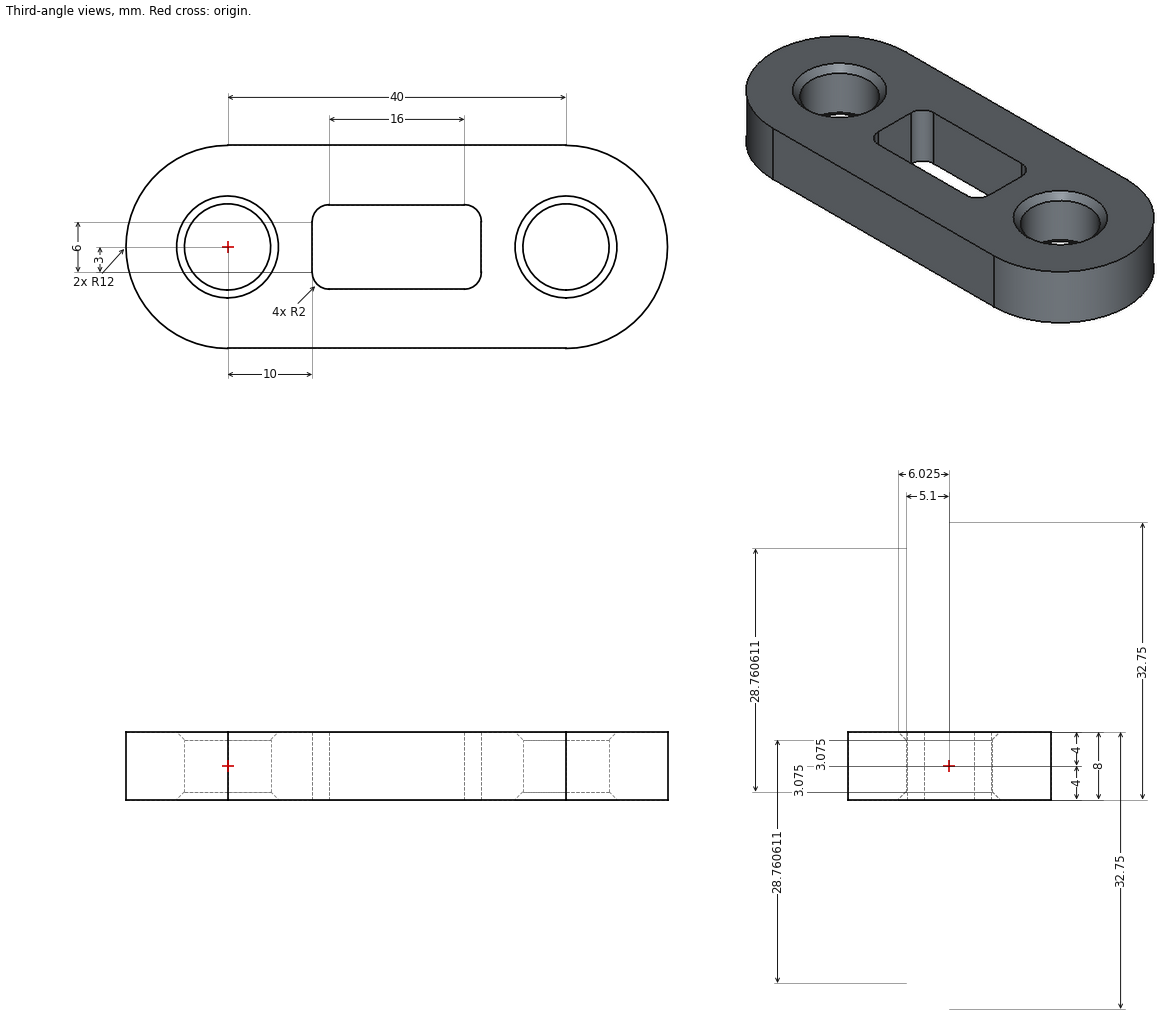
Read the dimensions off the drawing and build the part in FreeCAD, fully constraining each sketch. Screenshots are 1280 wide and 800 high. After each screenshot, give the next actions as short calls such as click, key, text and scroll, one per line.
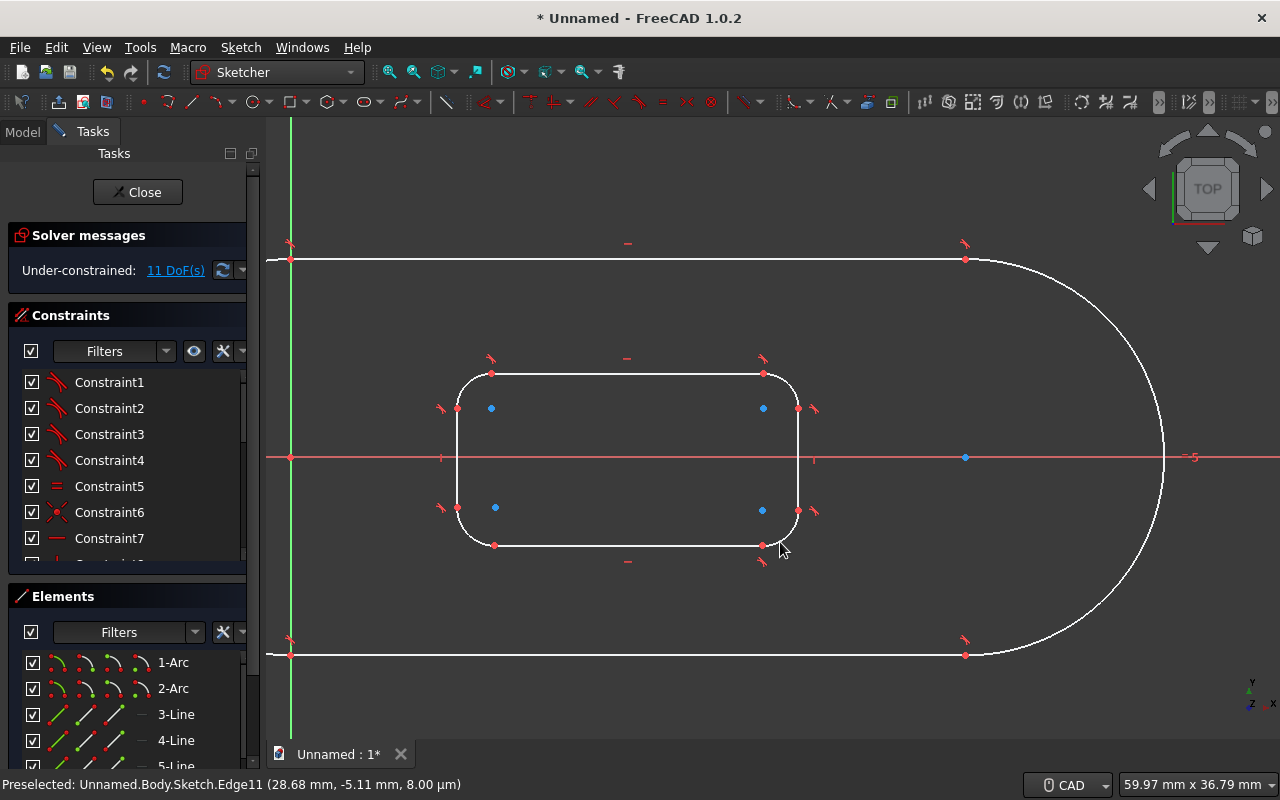
click(682, 546)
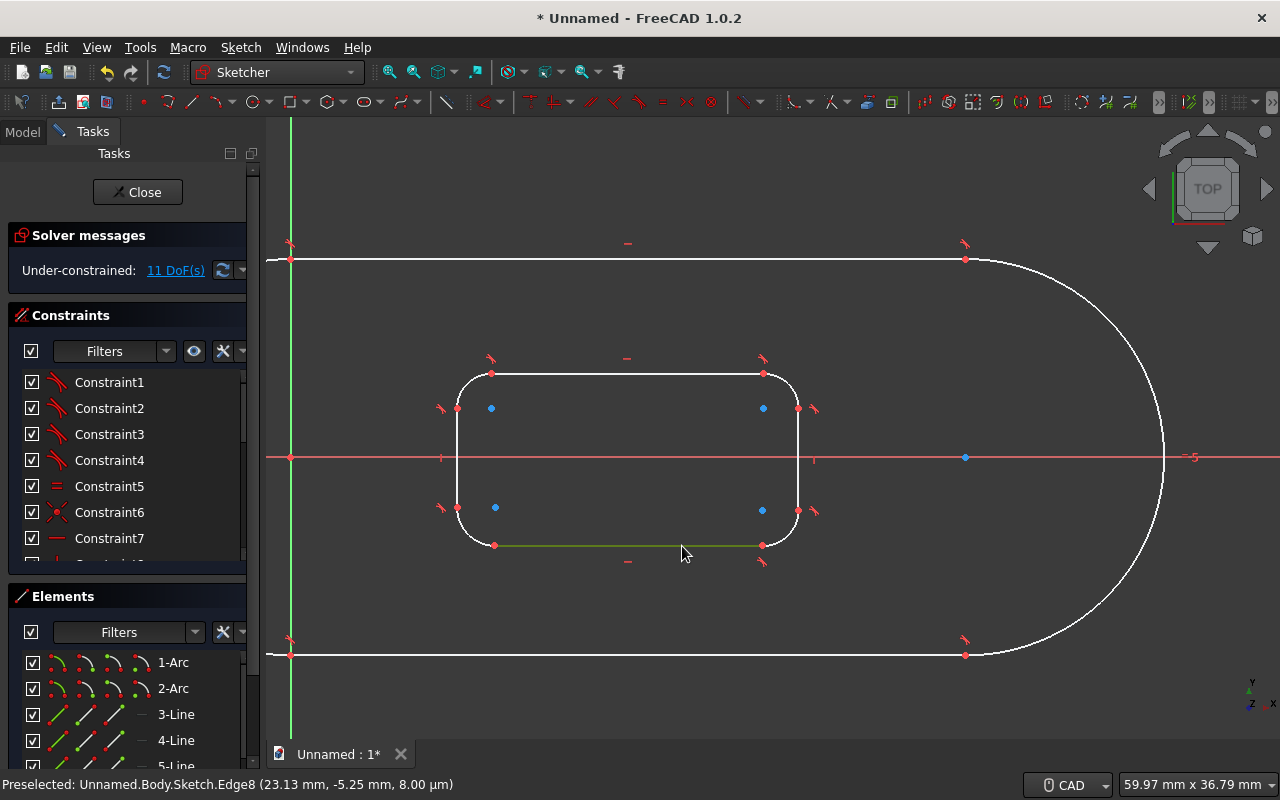
click(461, 524)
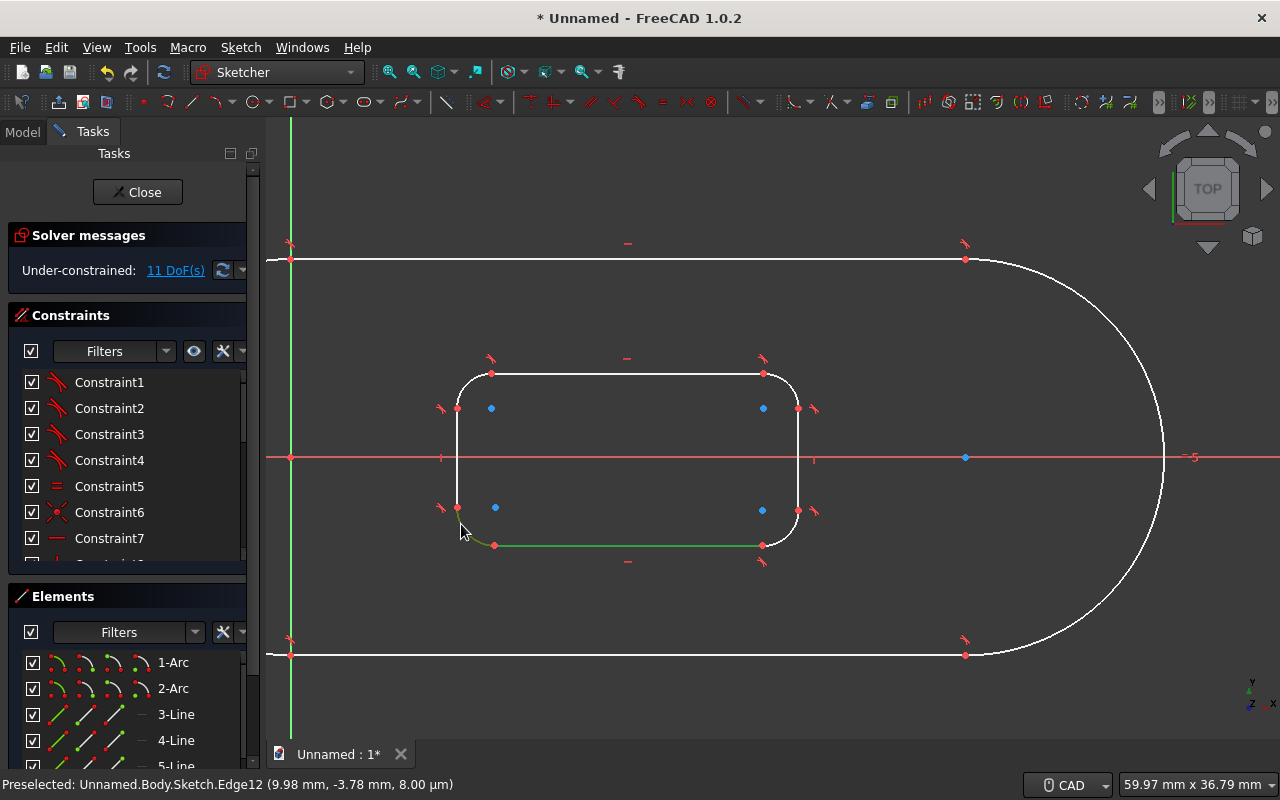
key(t)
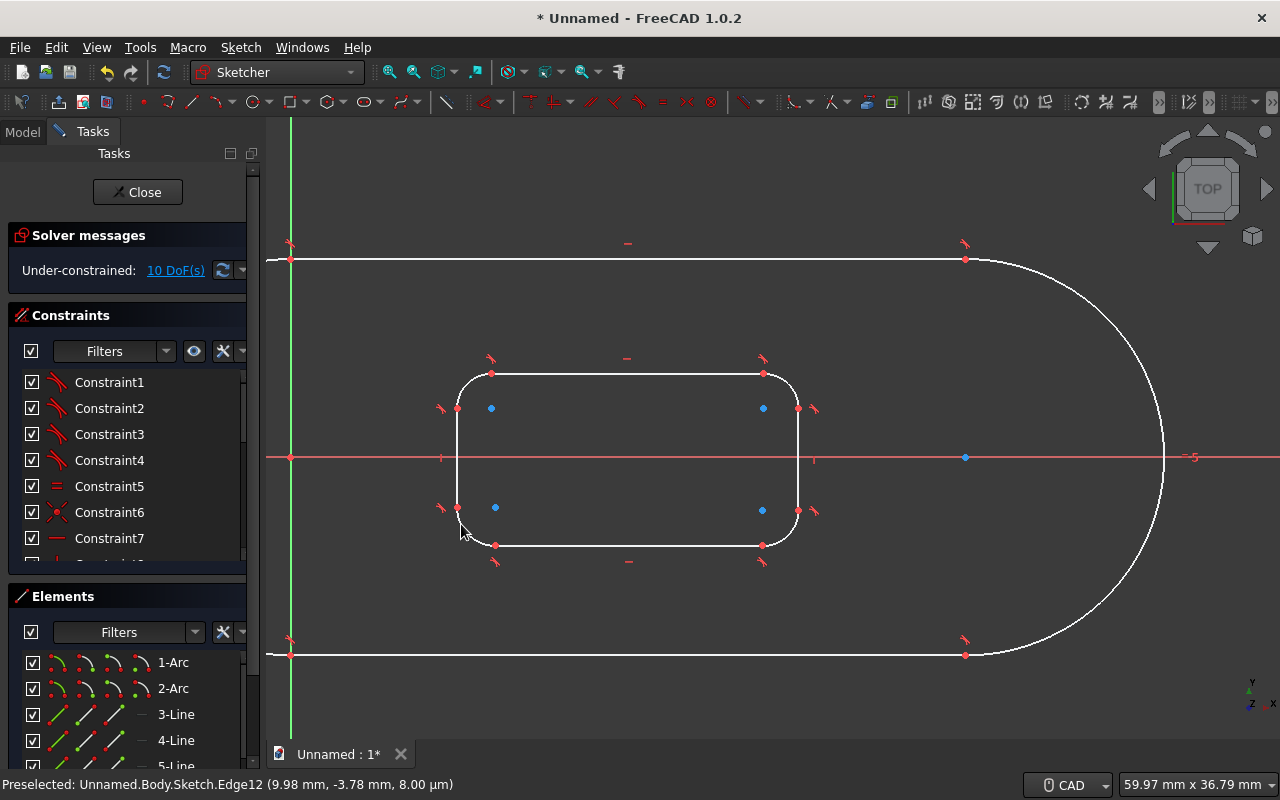
click(476, 378)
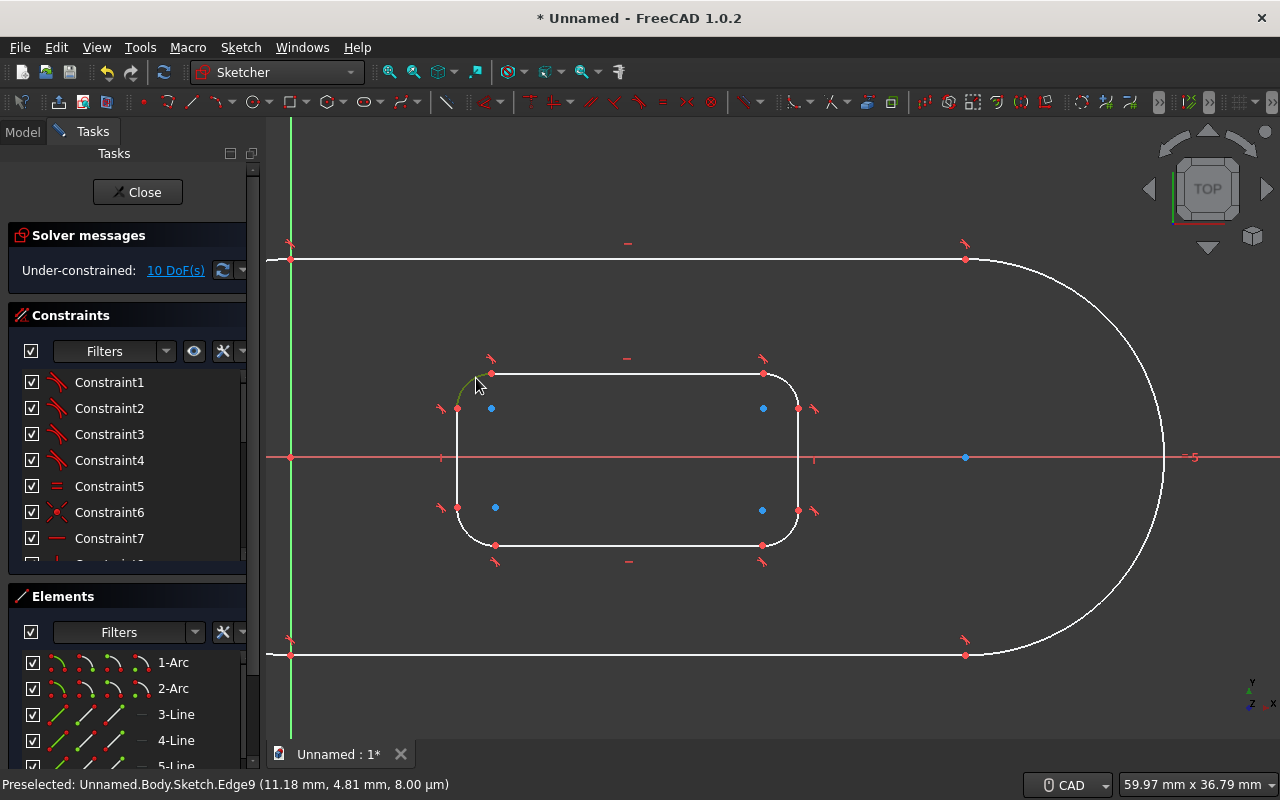
click(795, 393)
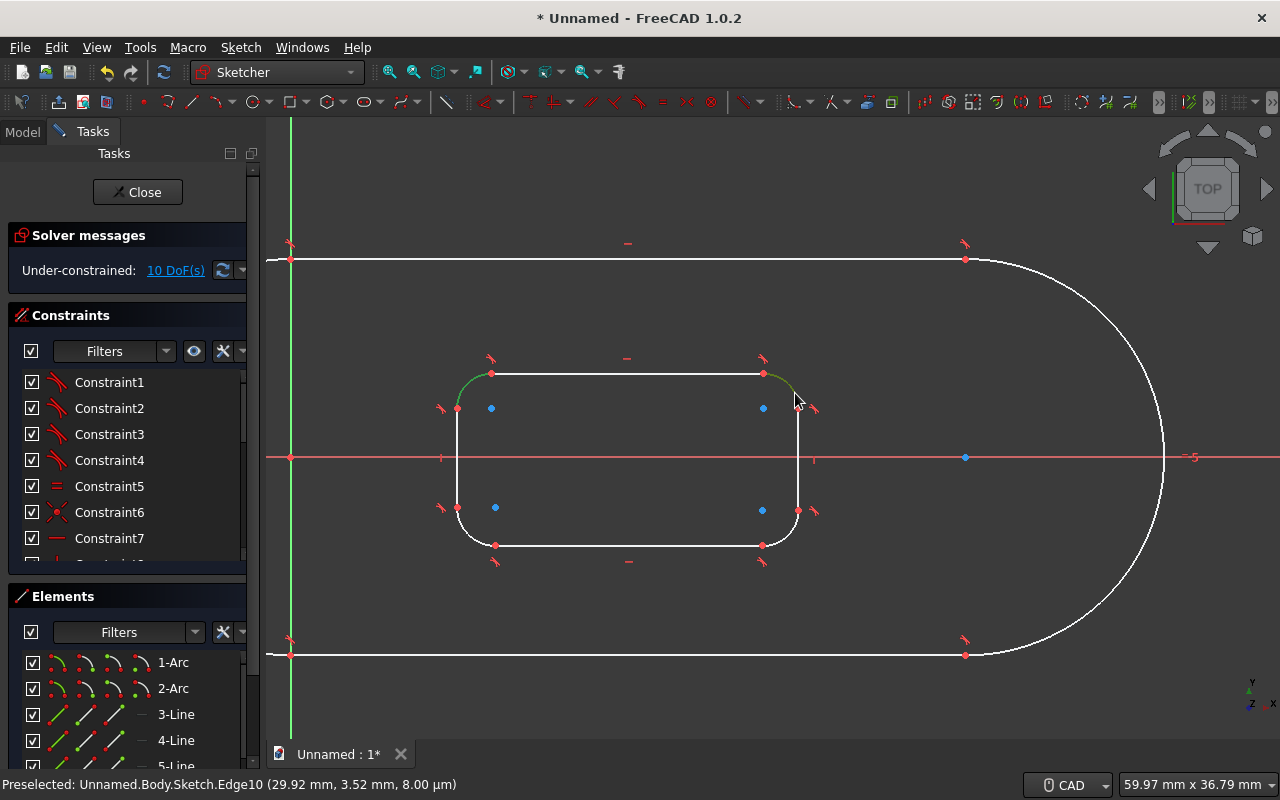
click(779, 542)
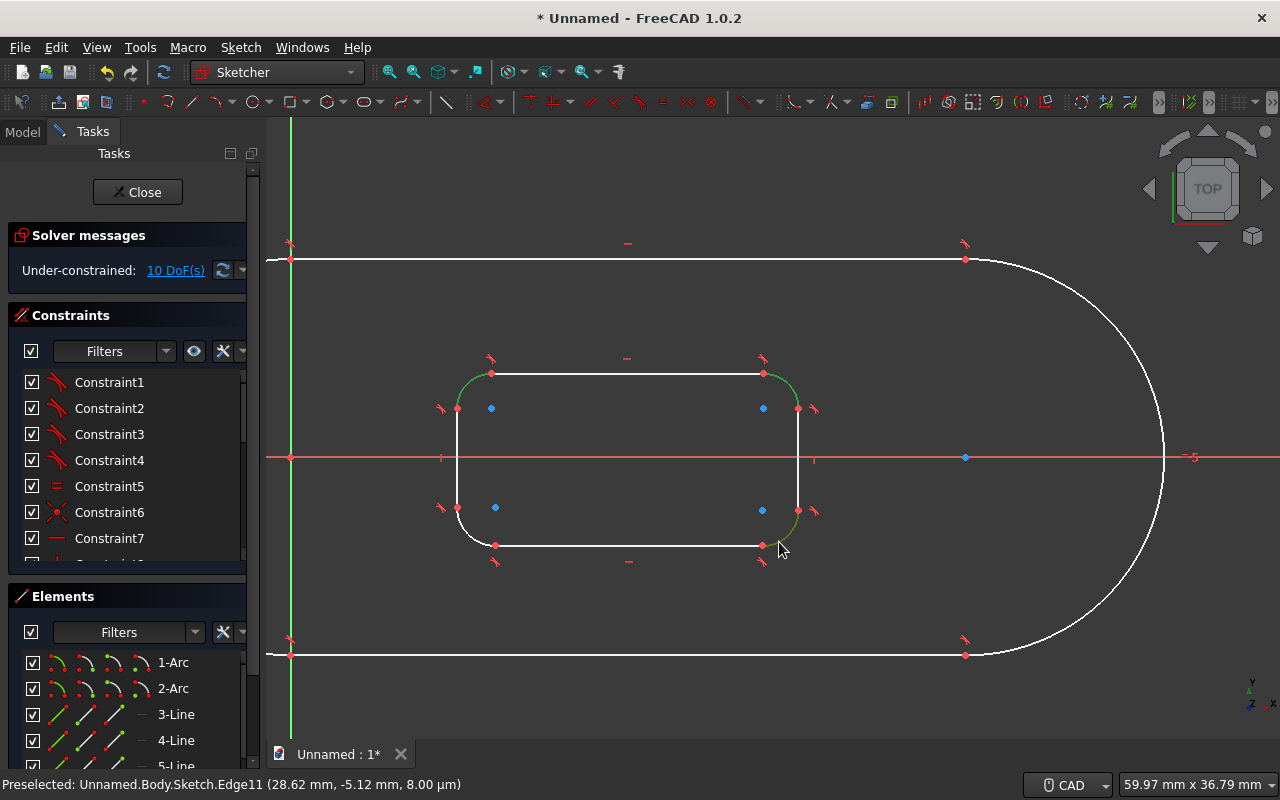
click(461, 525)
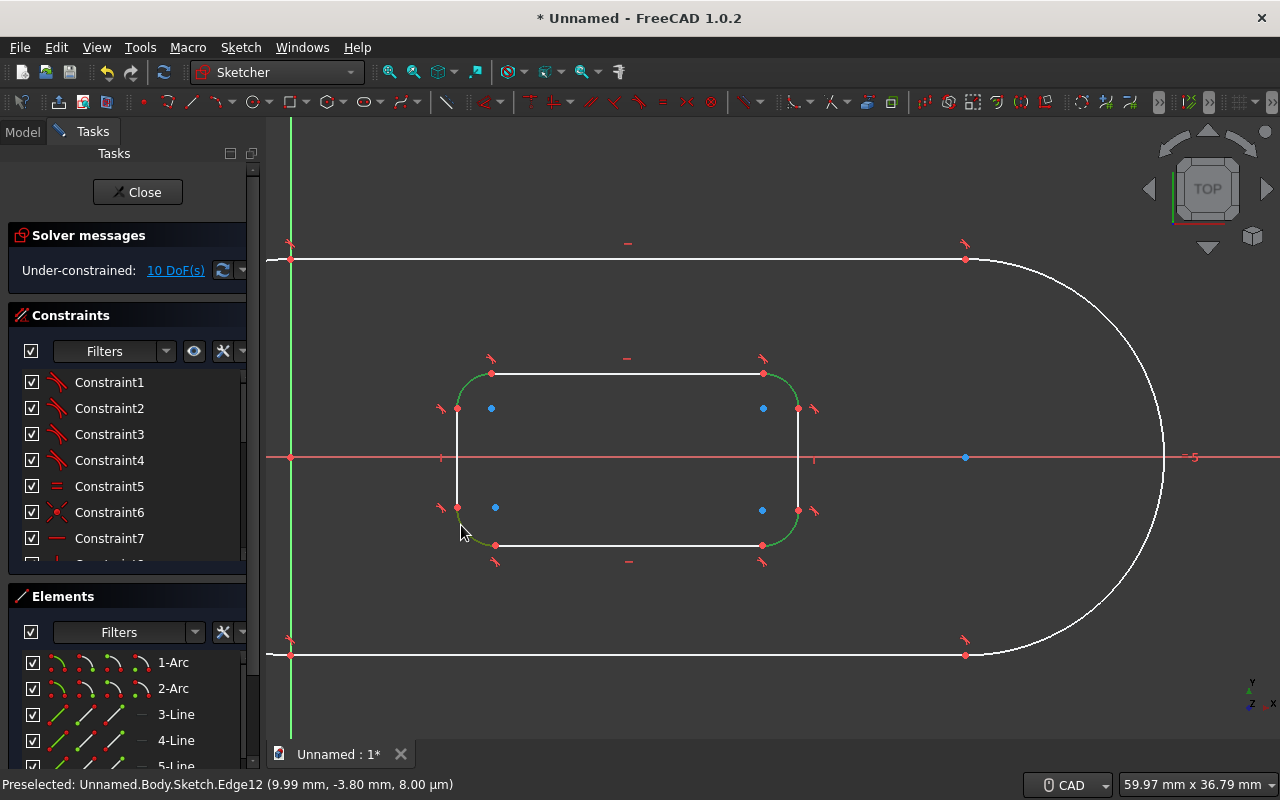
click(664, 102)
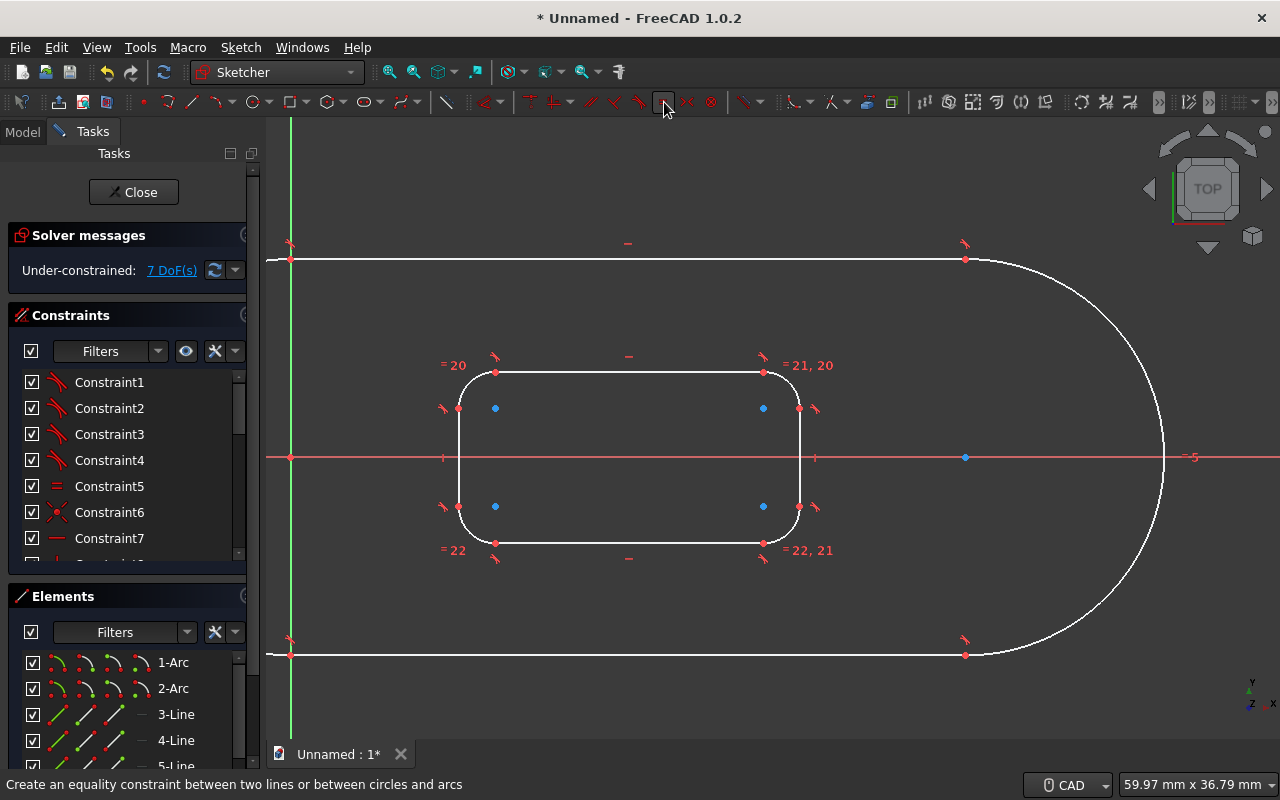
key(d)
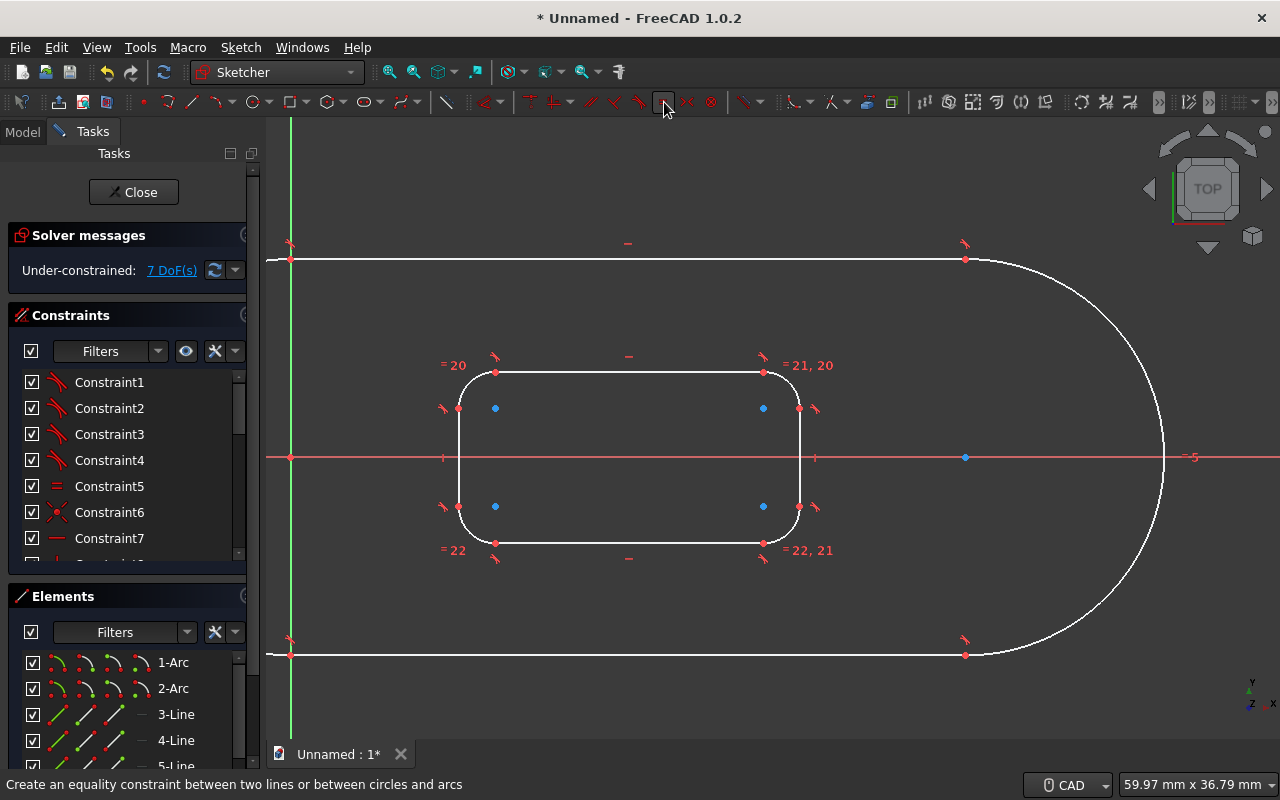
scroll(796, 392, down, 3)